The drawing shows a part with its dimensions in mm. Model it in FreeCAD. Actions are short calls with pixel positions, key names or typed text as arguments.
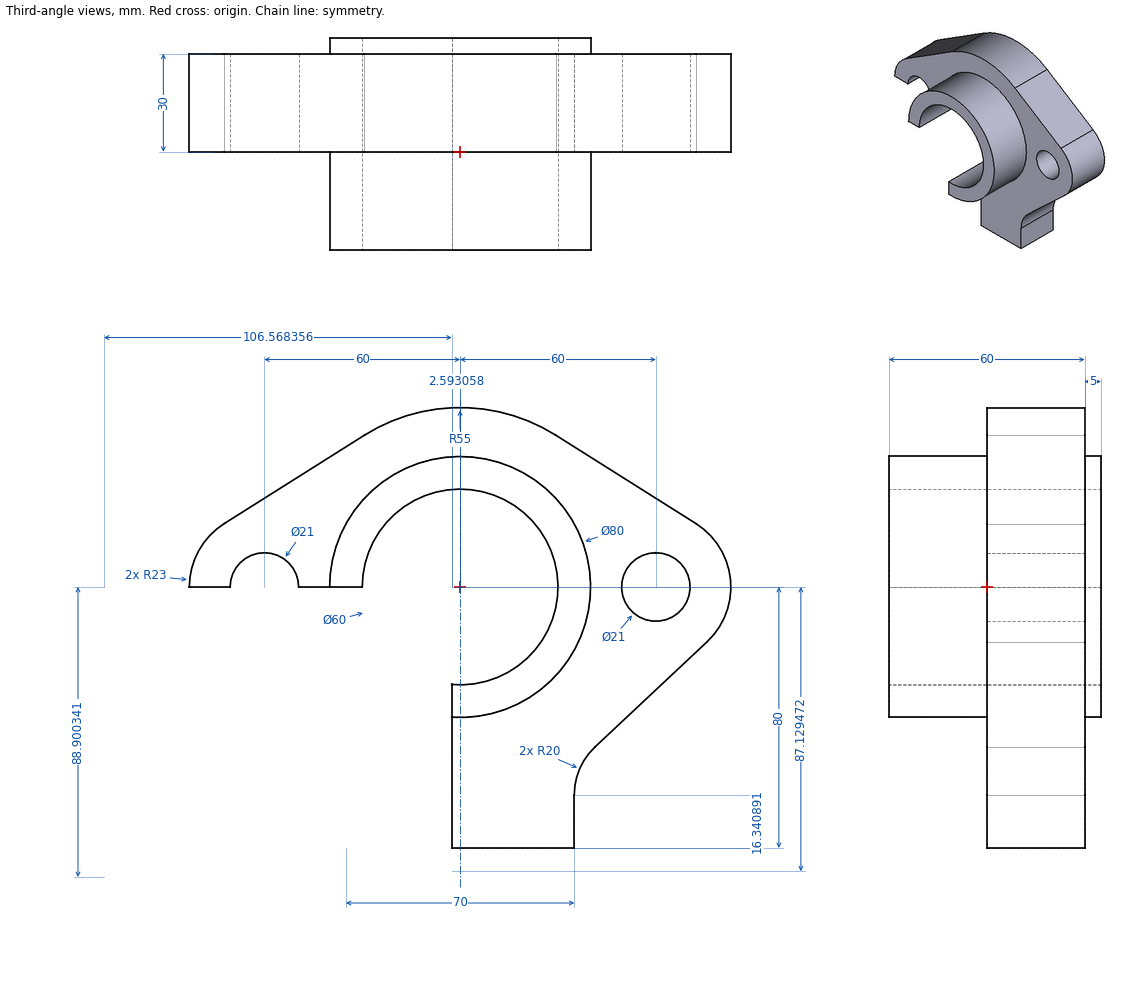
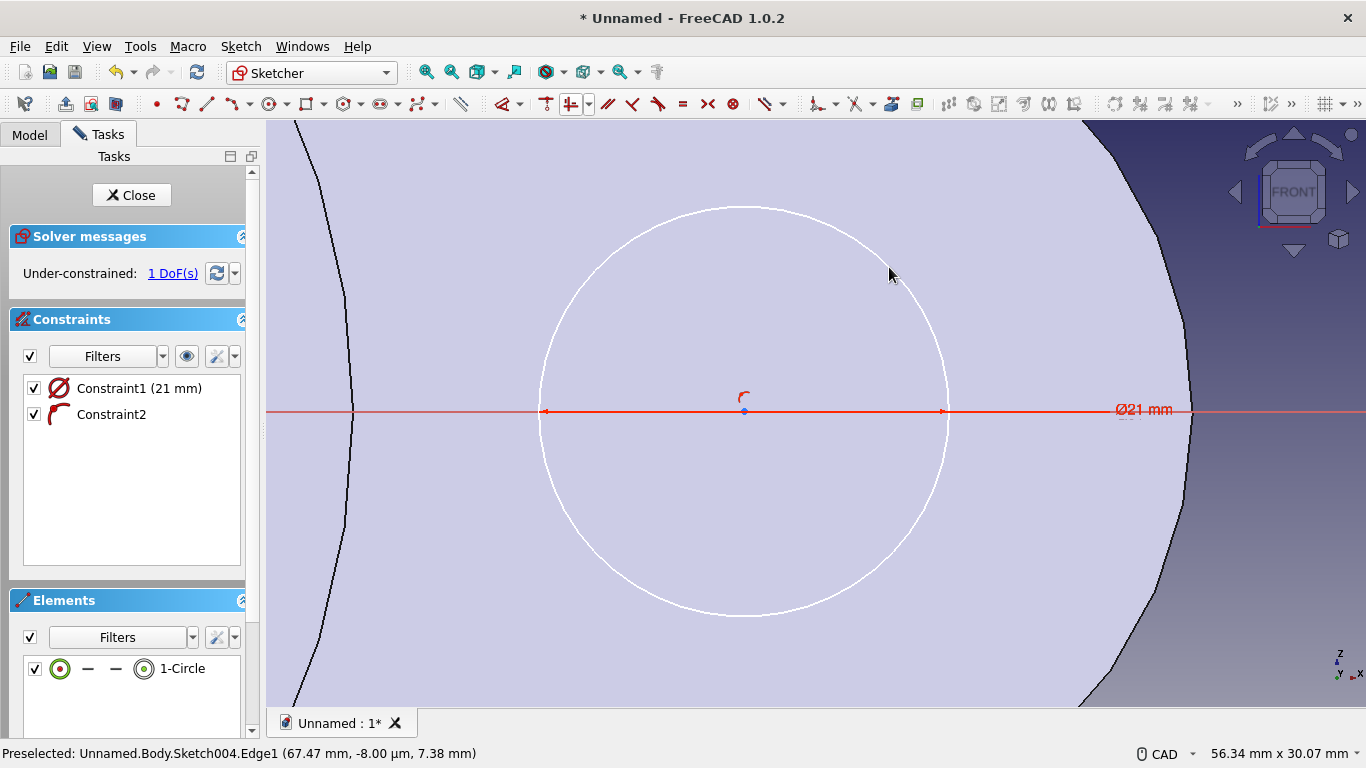
click(502, 104)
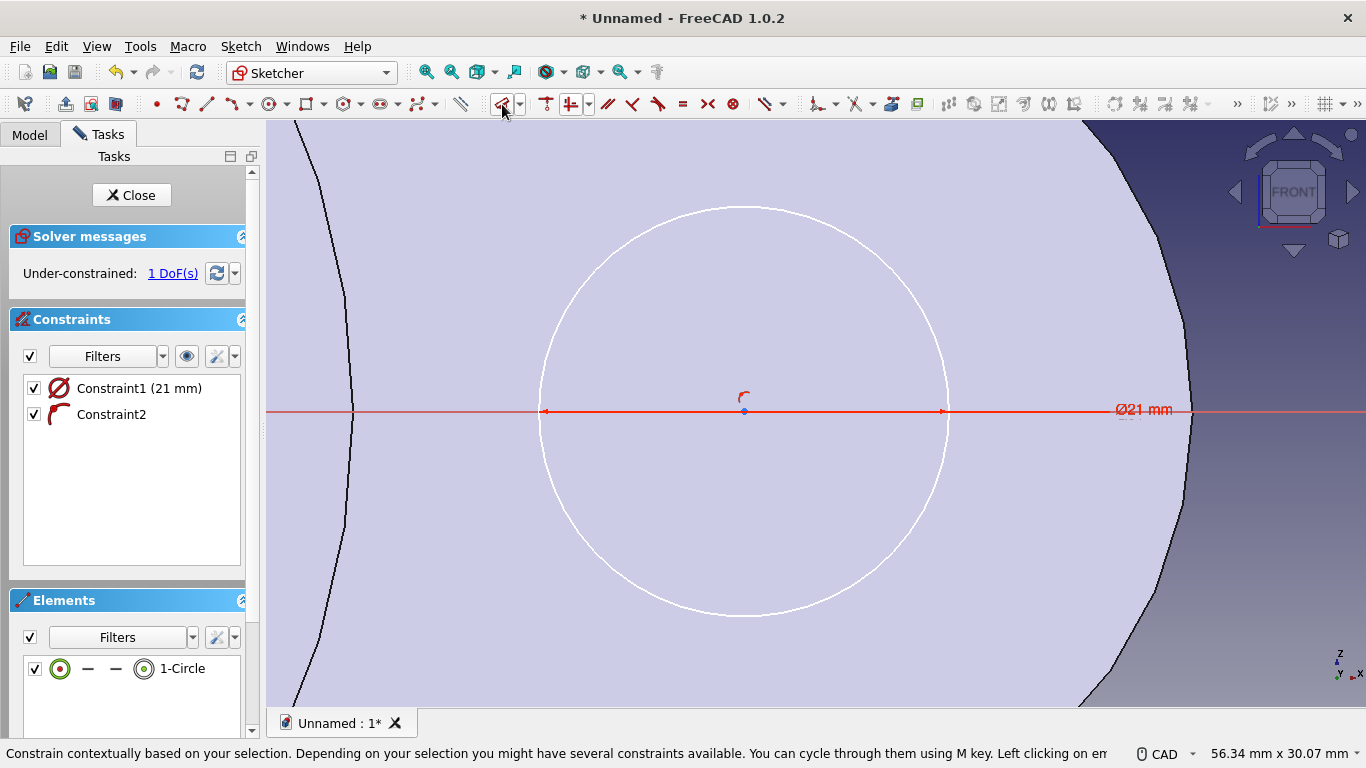
click(744, 412)
click(519, 446)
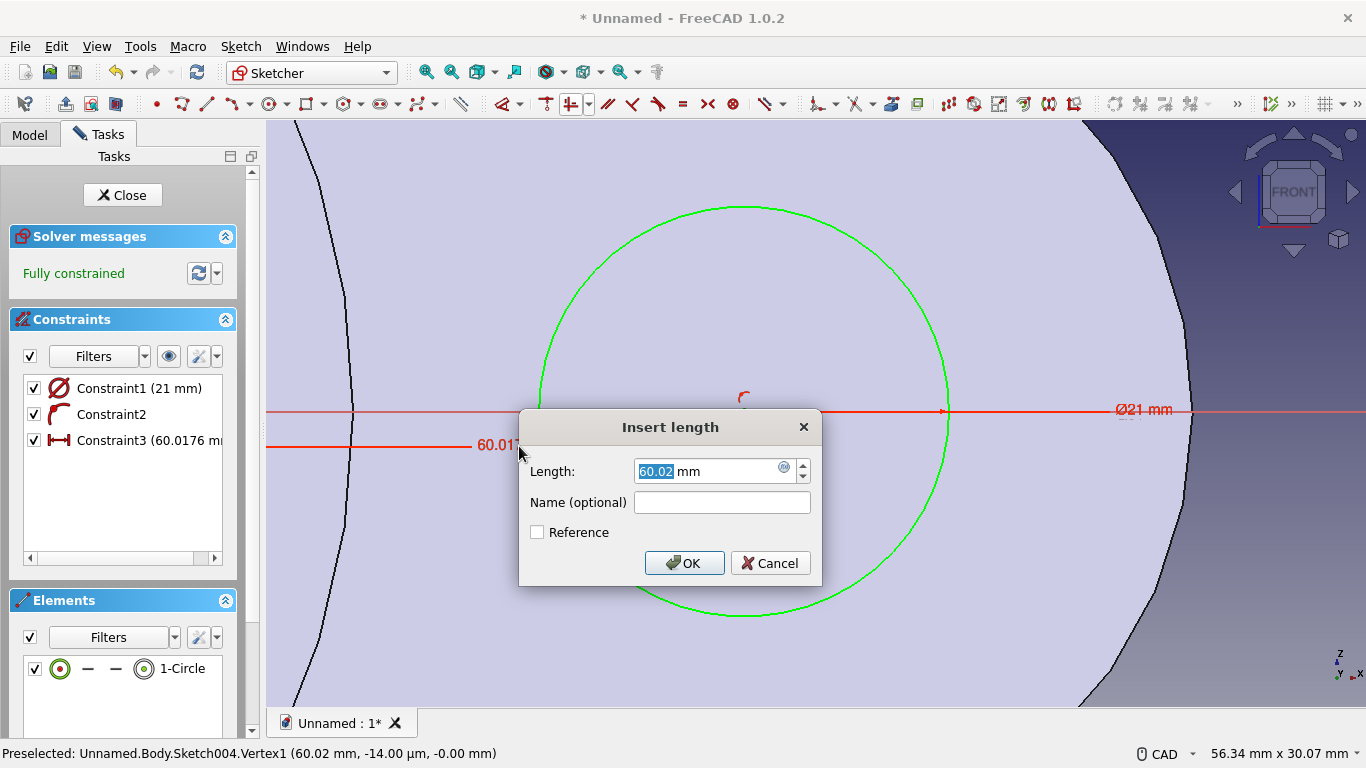
text(60)
key(Return)
key(Escape)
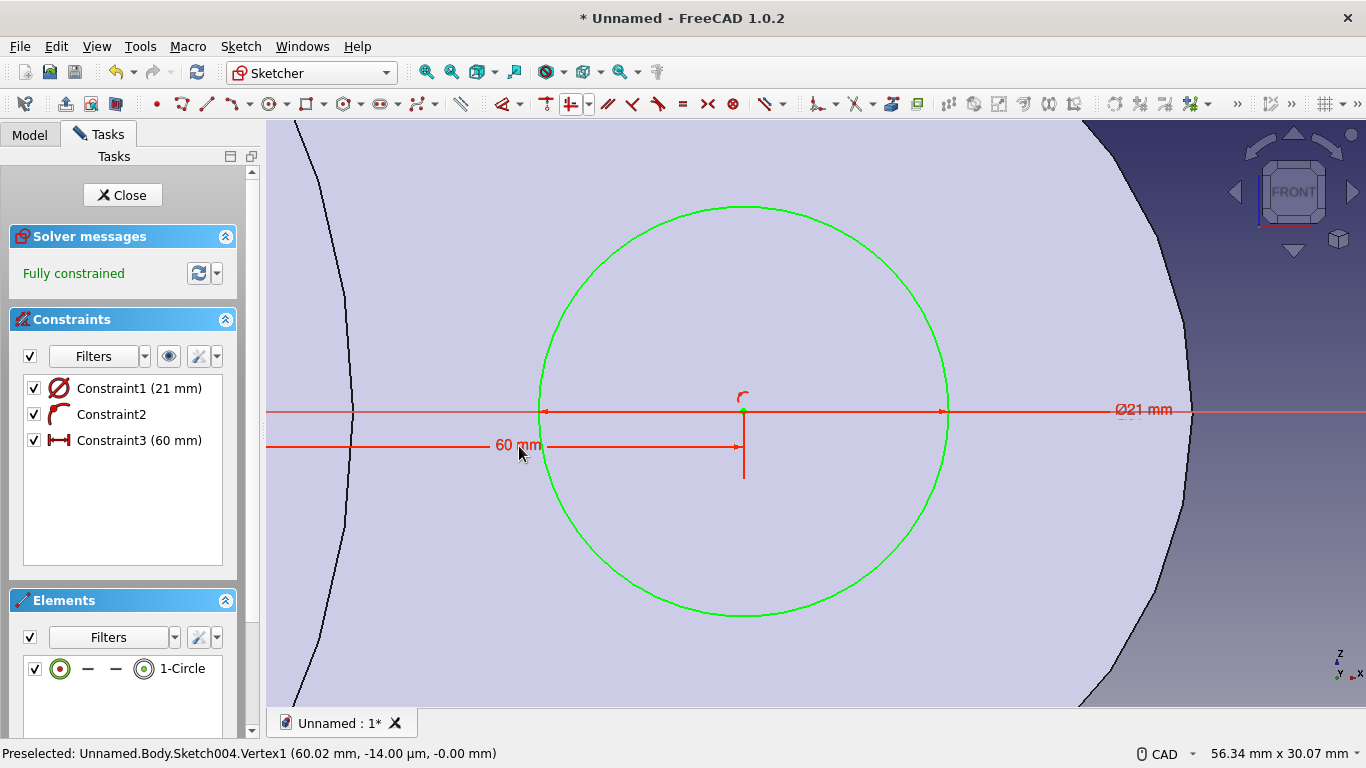
click(123, 195)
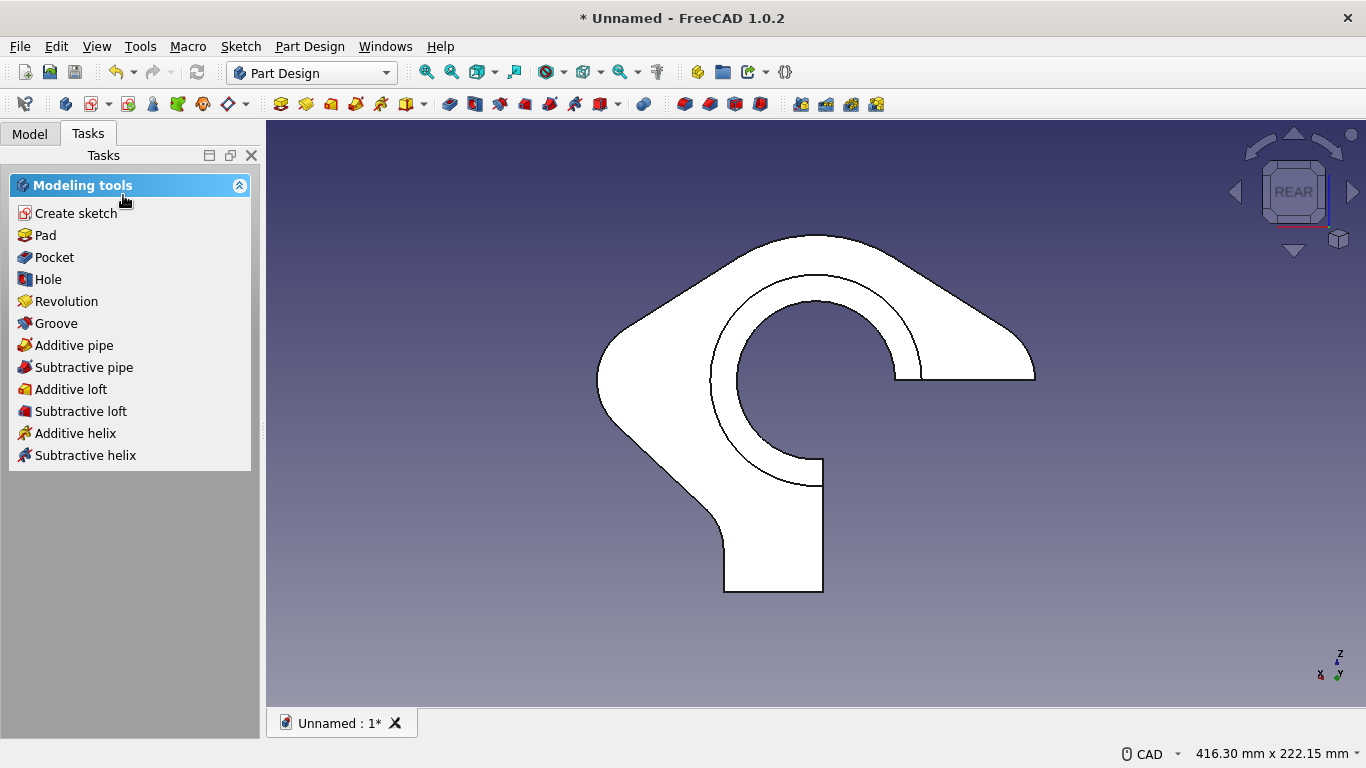
click(450, 104)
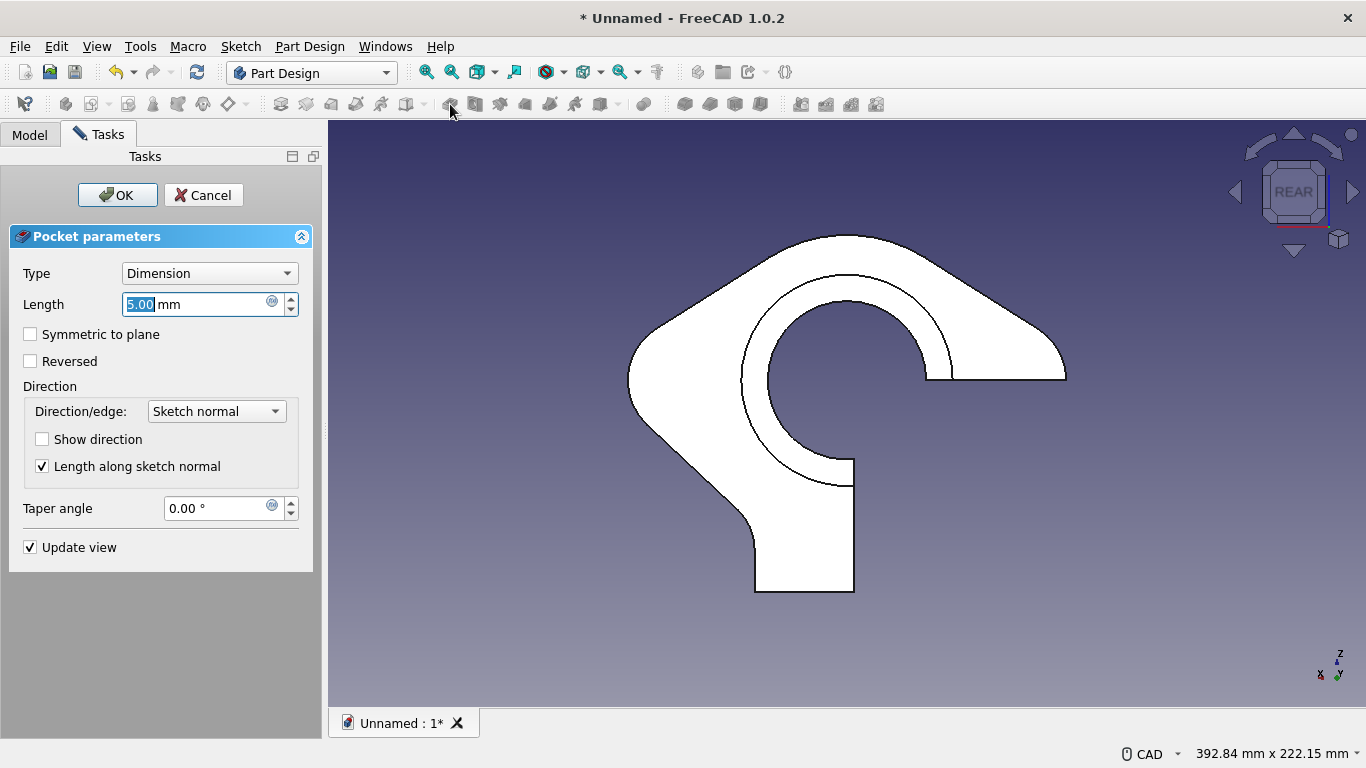
click(210, 274)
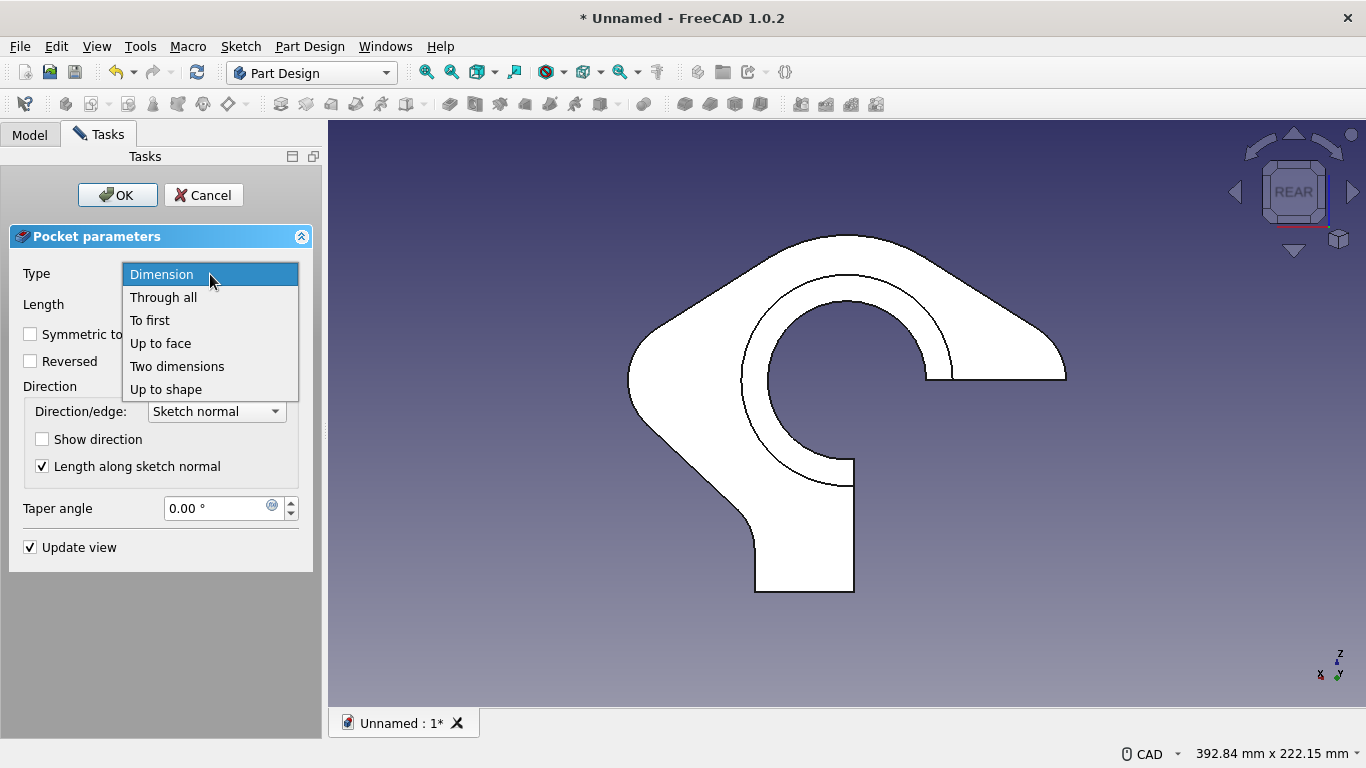
click(208, 366)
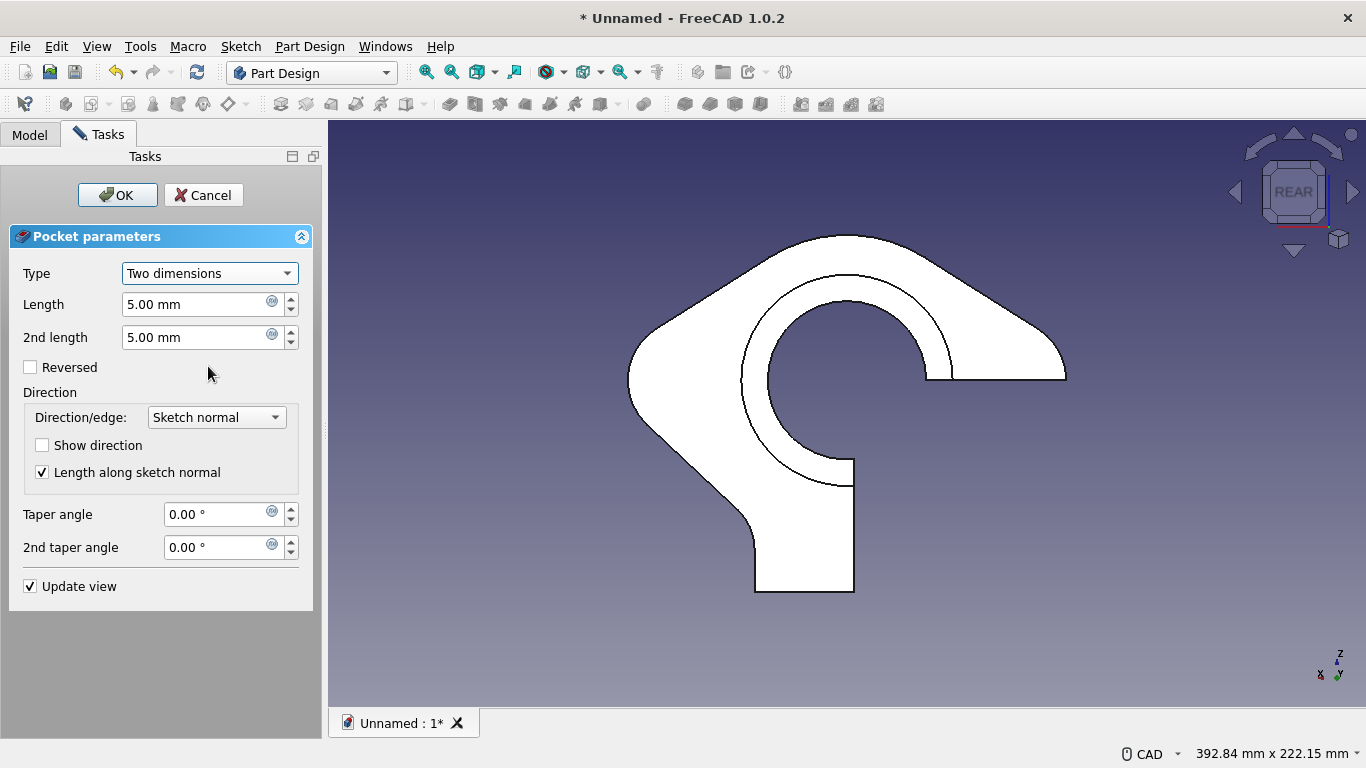
triple_click(204, 304)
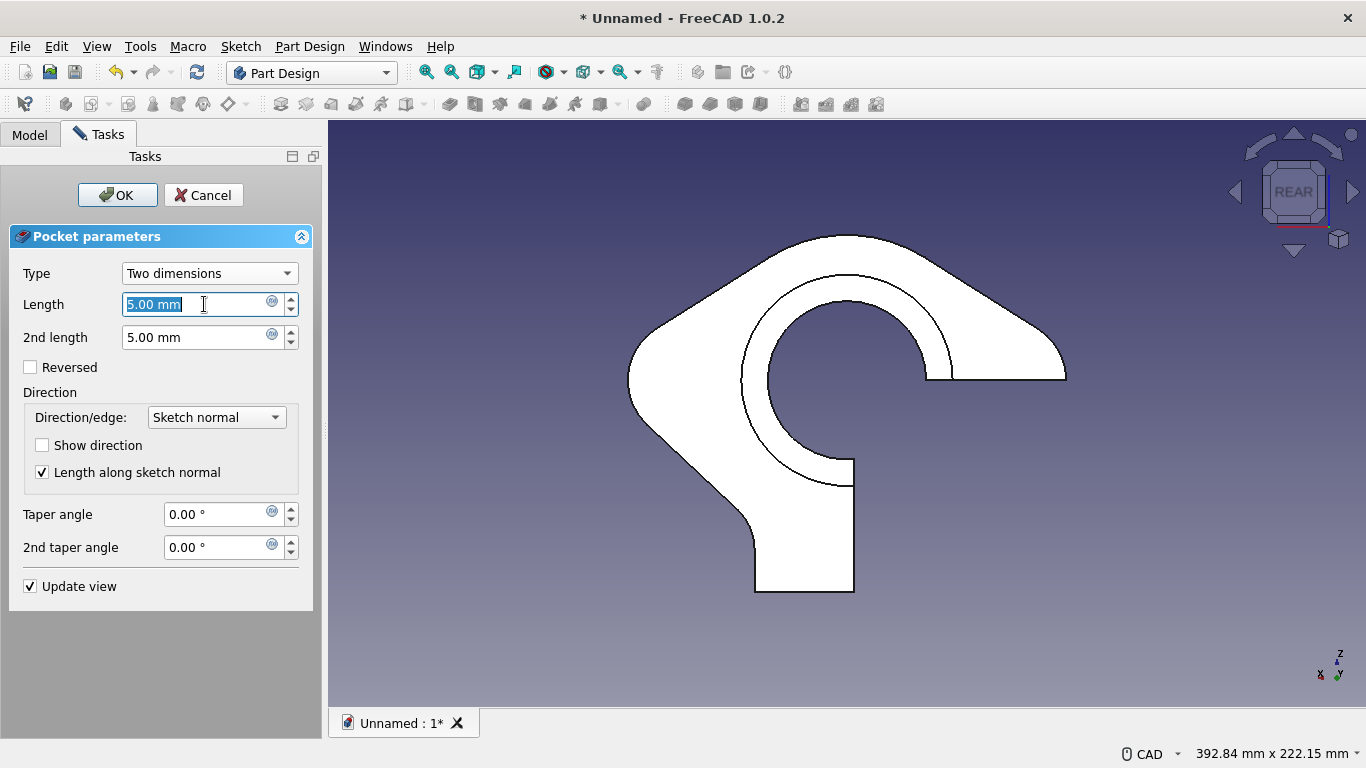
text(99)
key(Tab)